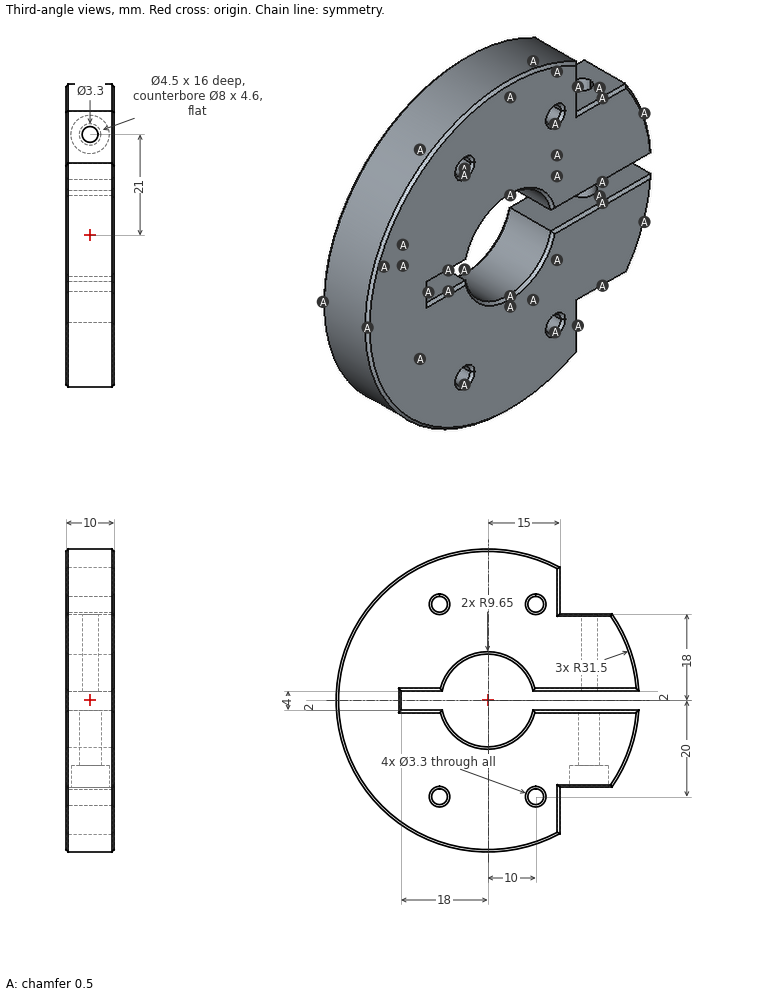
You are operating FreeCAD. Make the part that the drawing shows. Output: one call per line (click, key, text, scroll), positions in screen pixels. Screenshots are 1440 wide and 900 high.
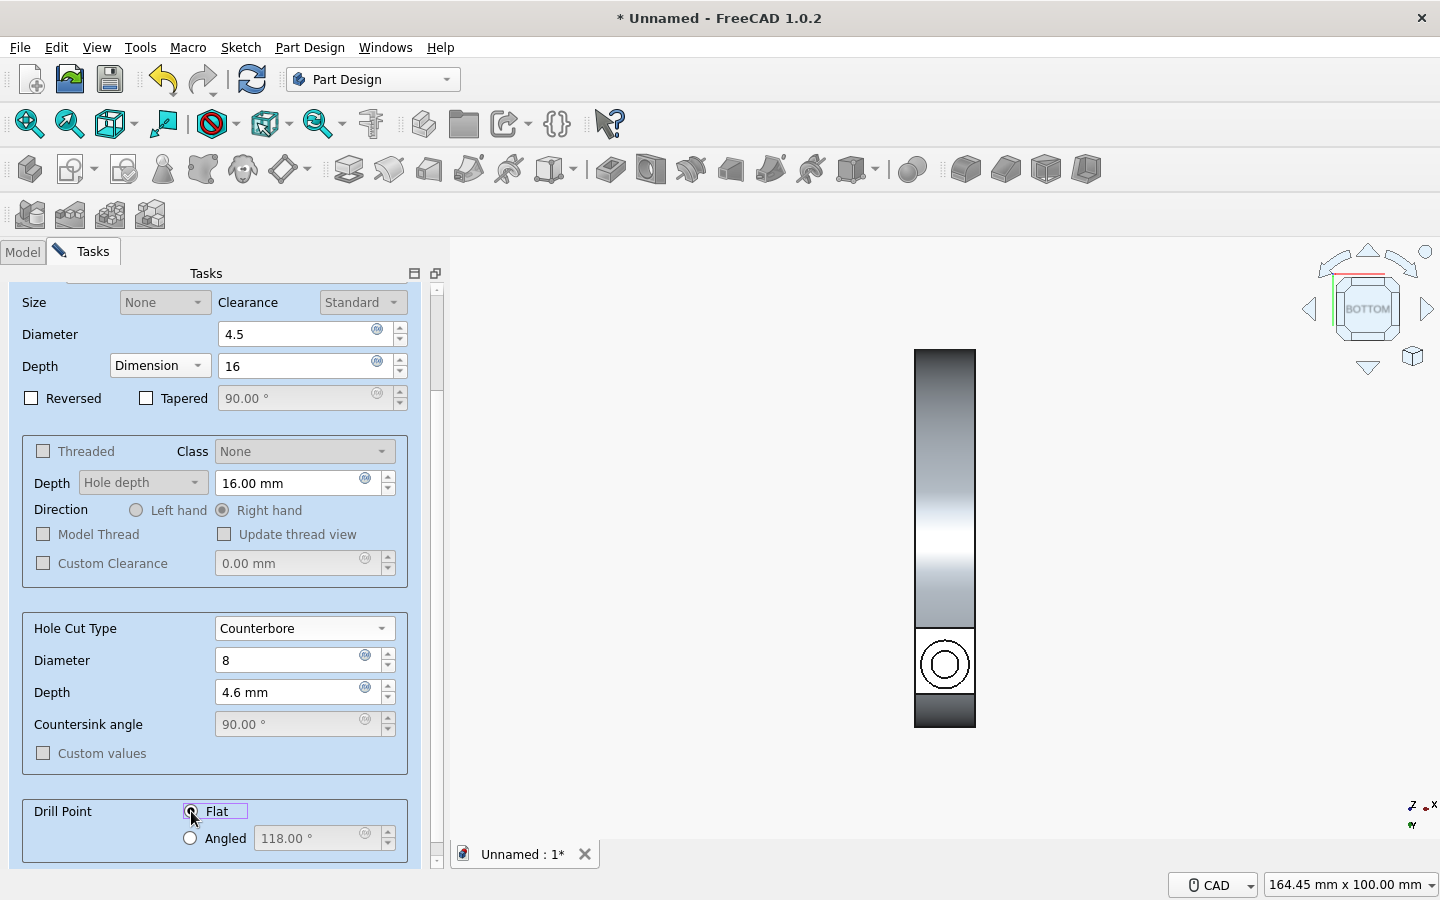
scroll(437, 576, up, 3)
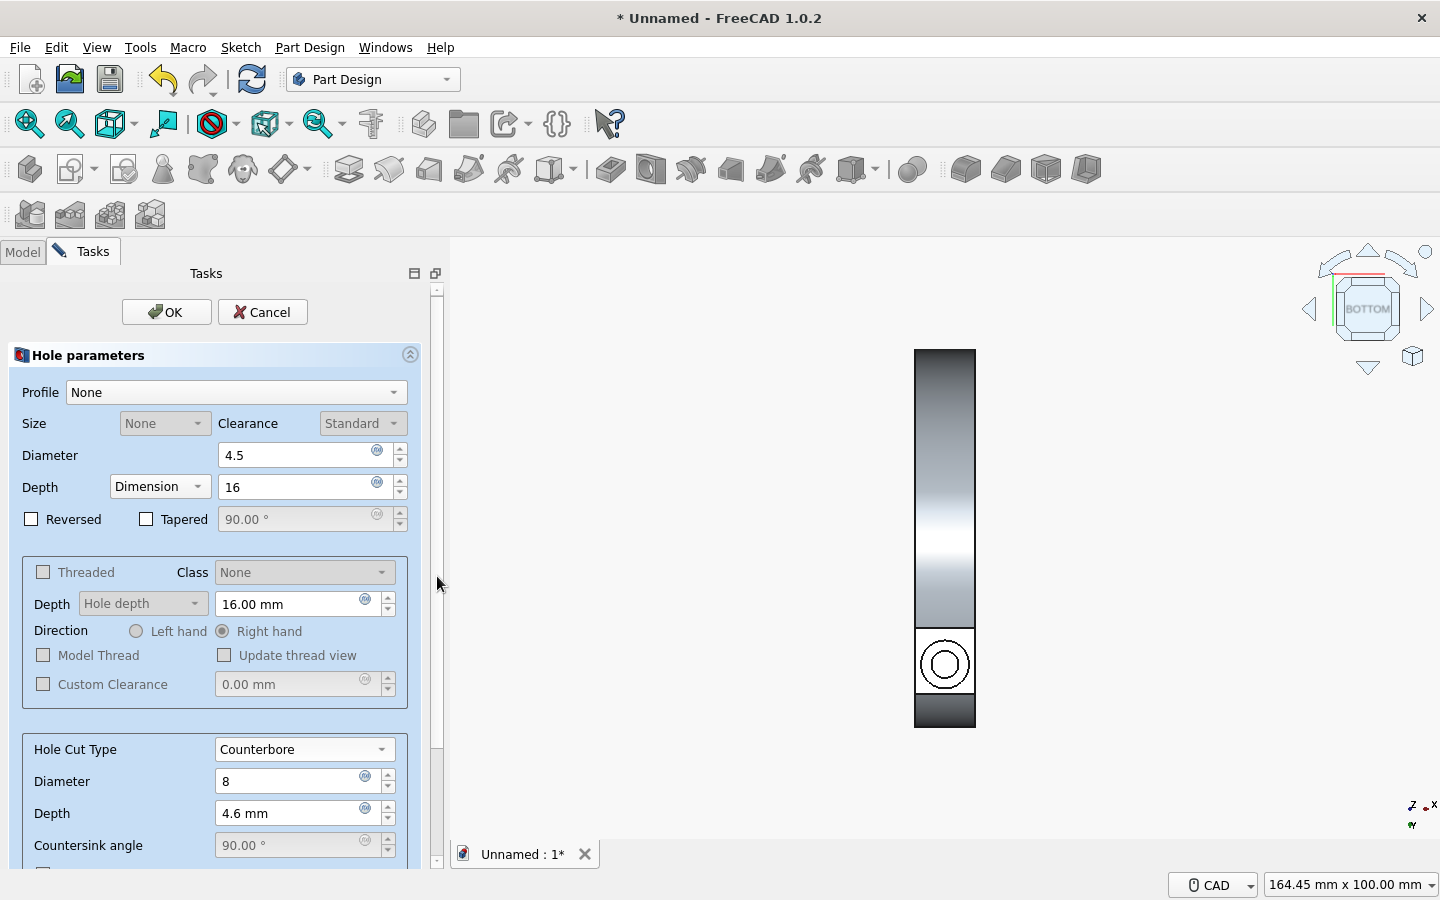
click(167, 312)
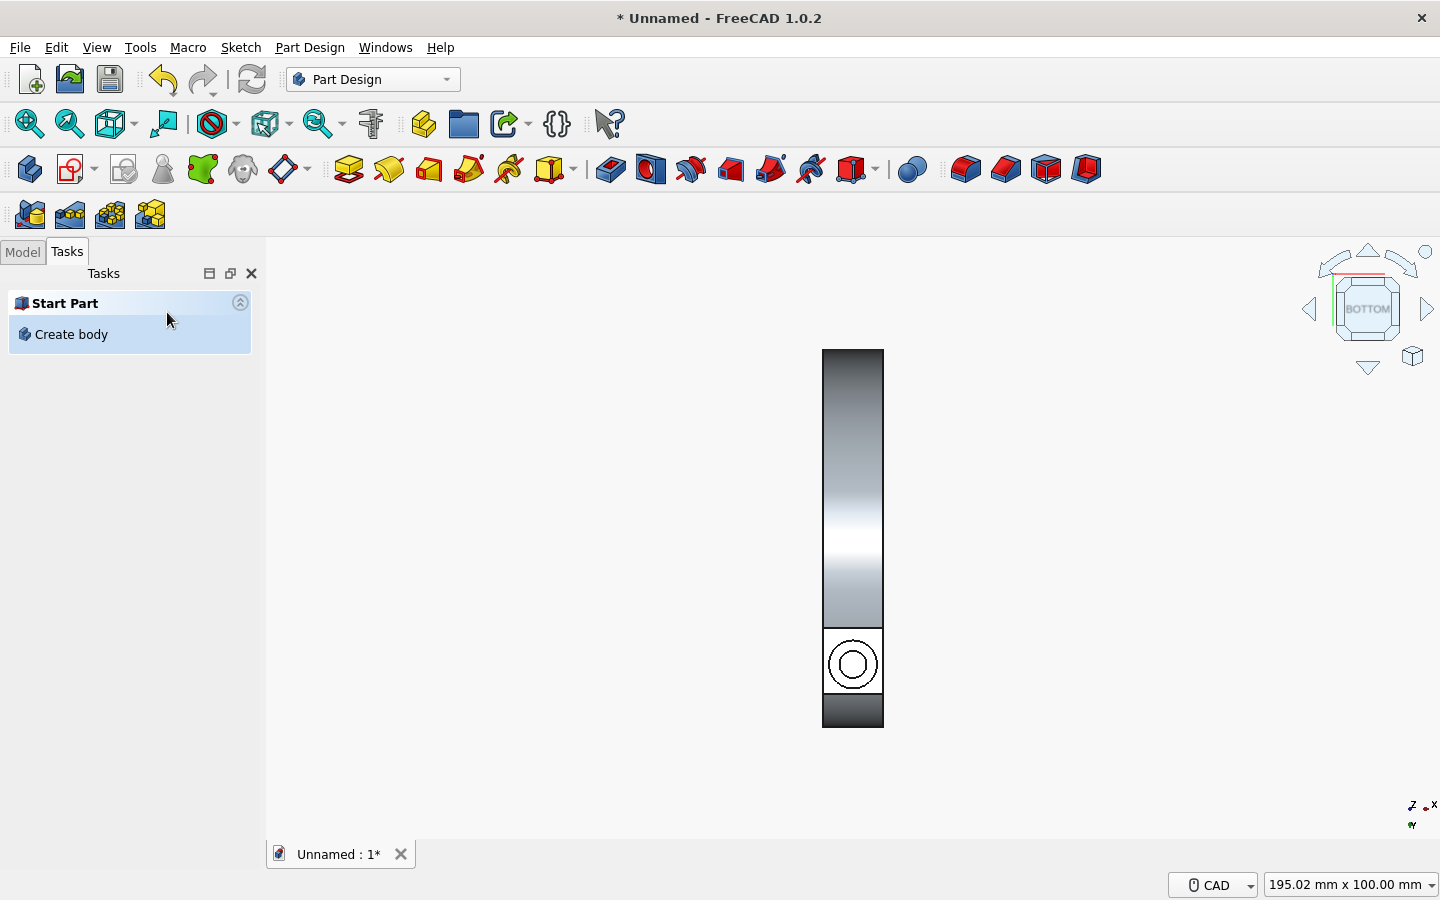
click(853, 660)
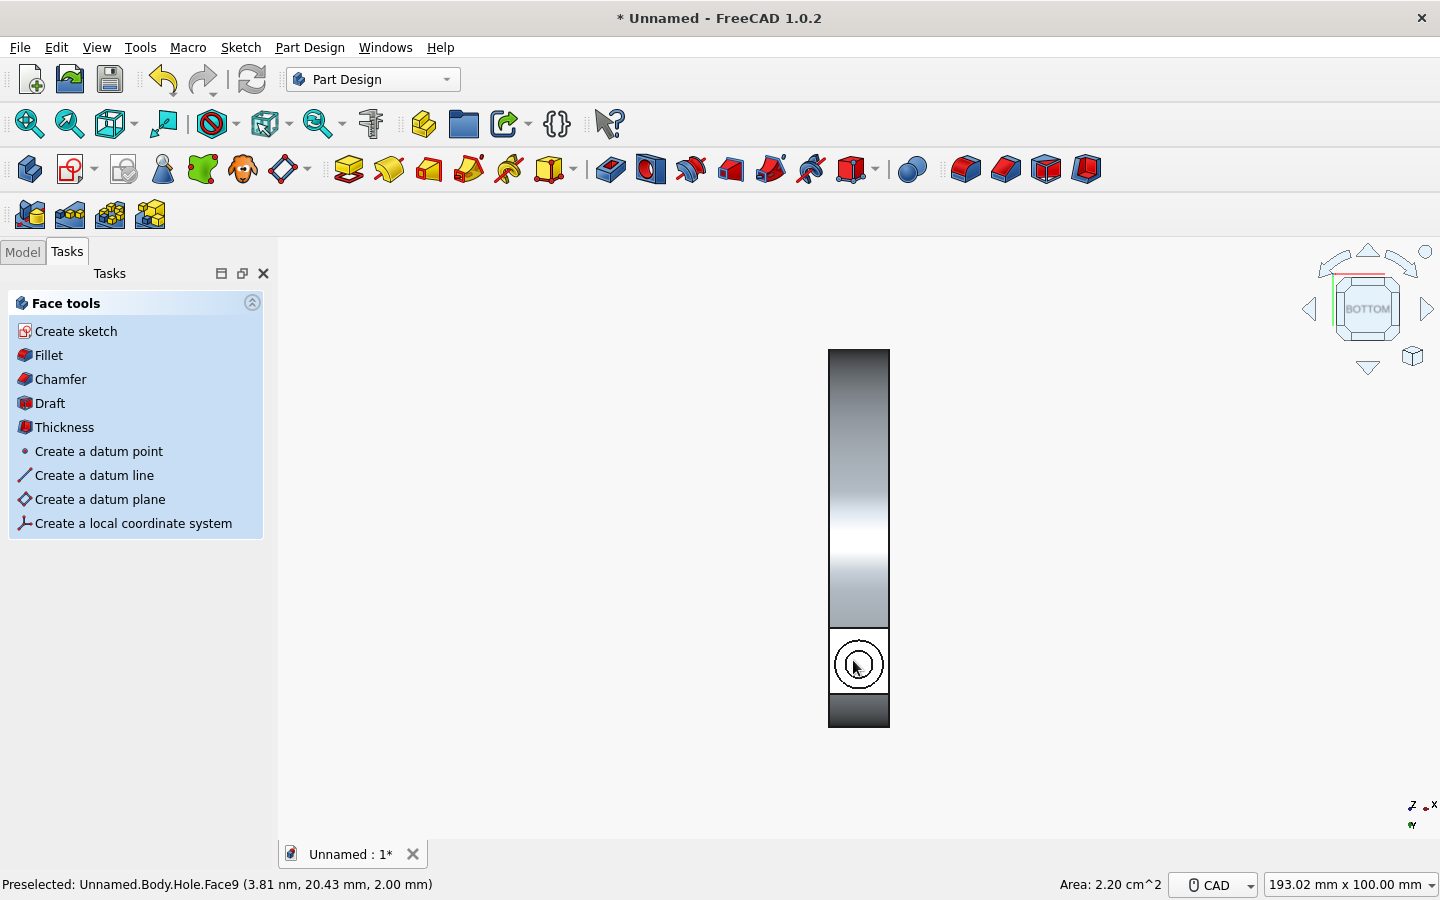
click(70, 170)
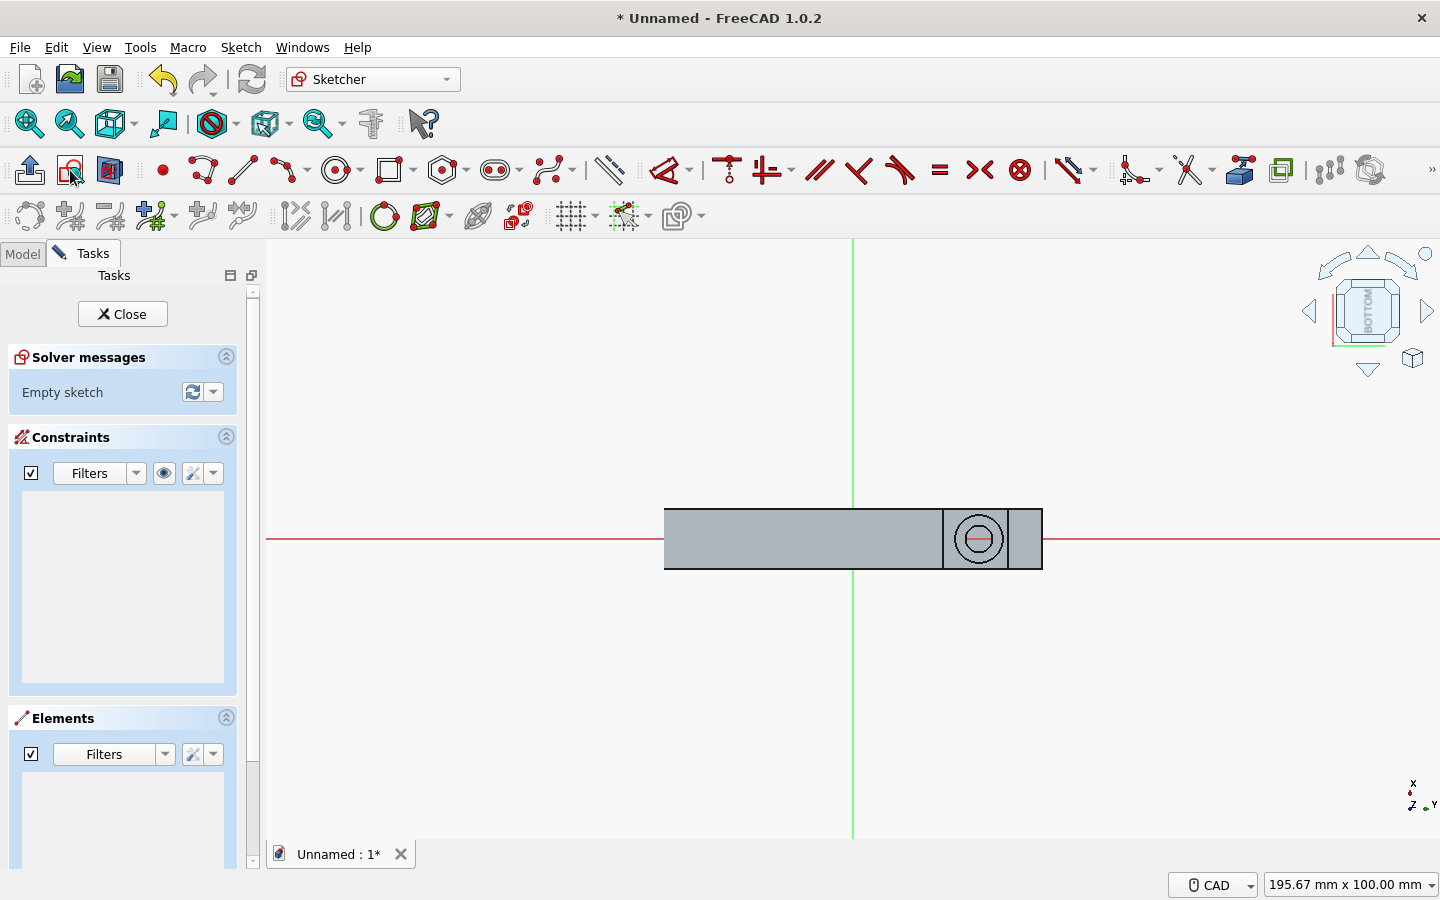
scroll(989, 539, up, 15)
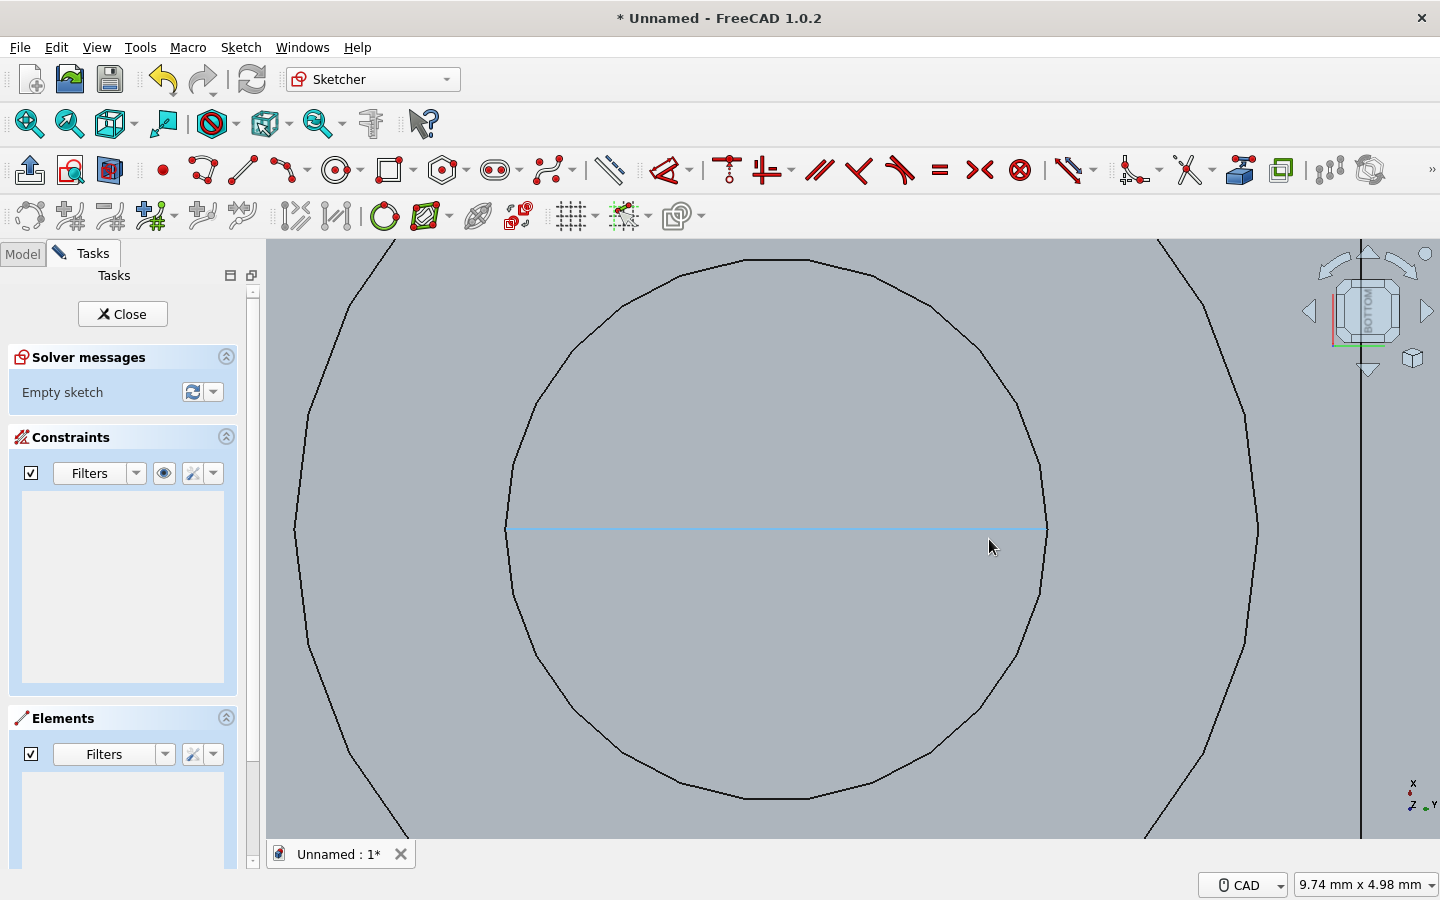
key(g)
key(c)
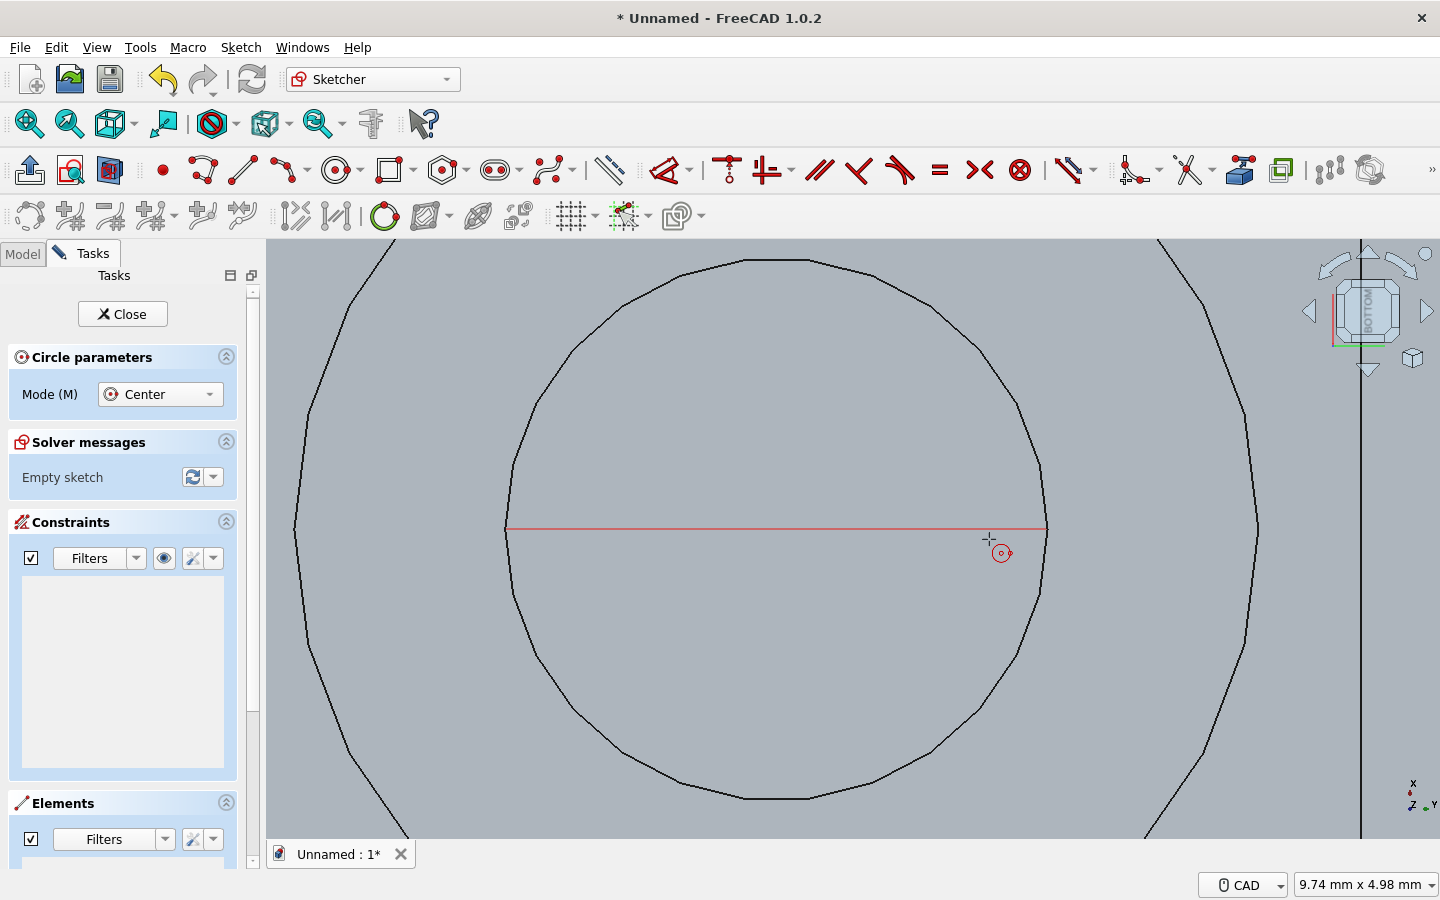
click(776, 529)
click(917, 389)
key(Escape)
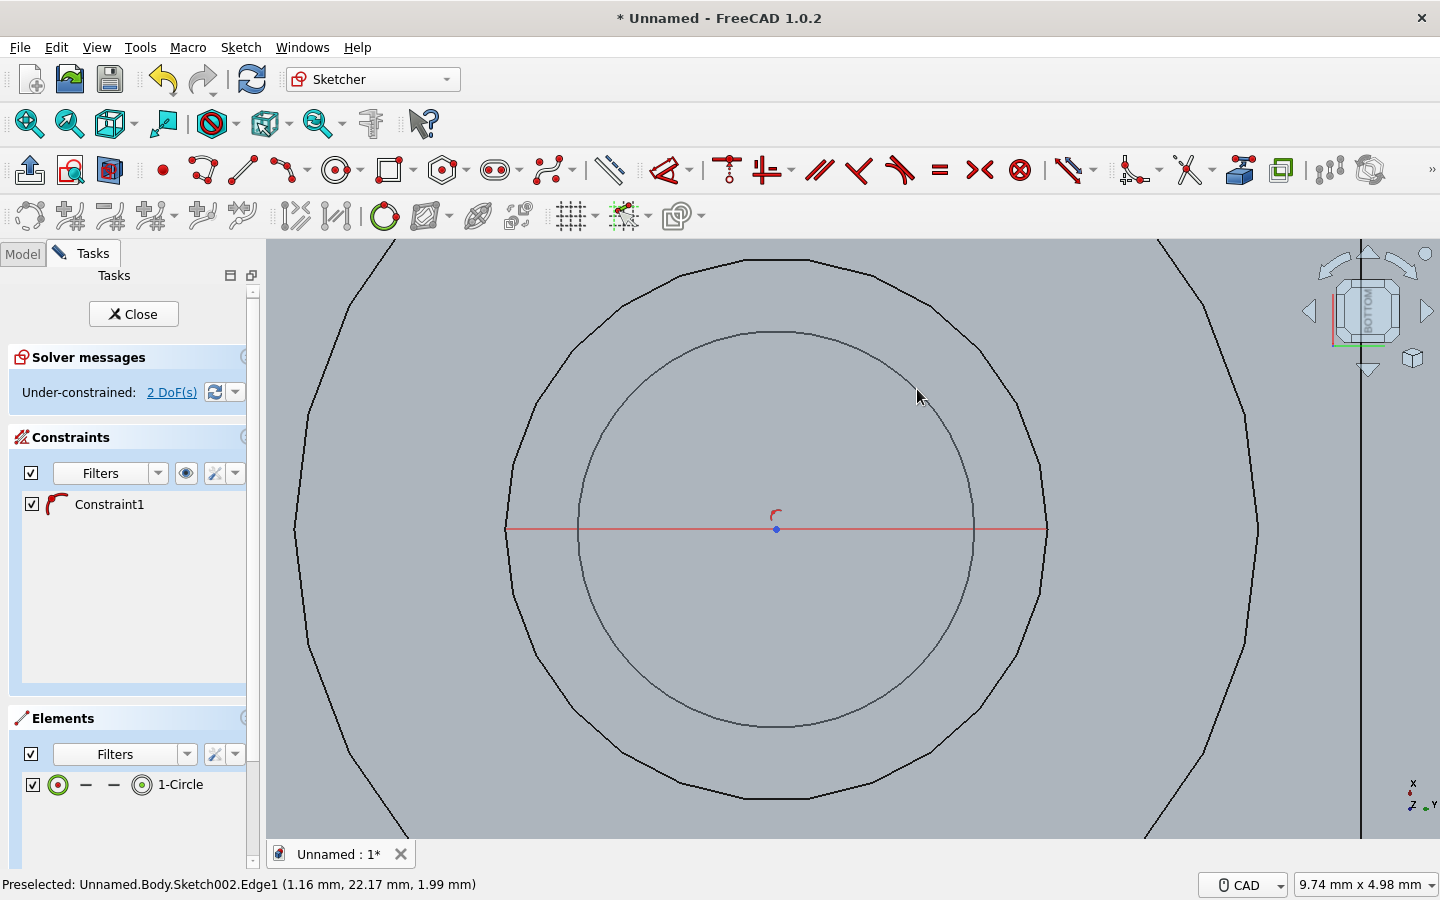
click(664, 170)